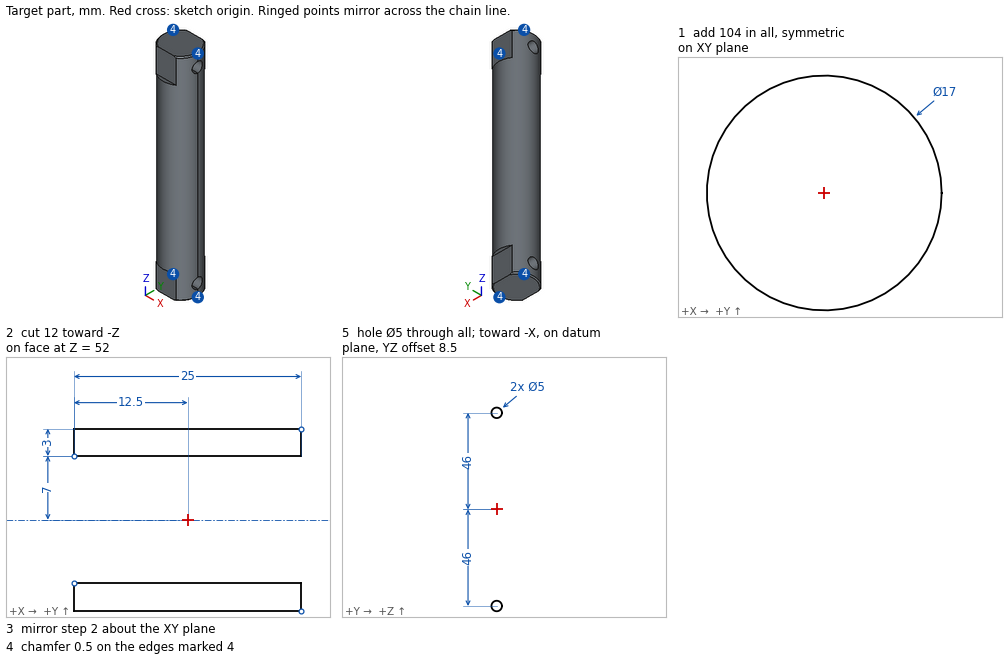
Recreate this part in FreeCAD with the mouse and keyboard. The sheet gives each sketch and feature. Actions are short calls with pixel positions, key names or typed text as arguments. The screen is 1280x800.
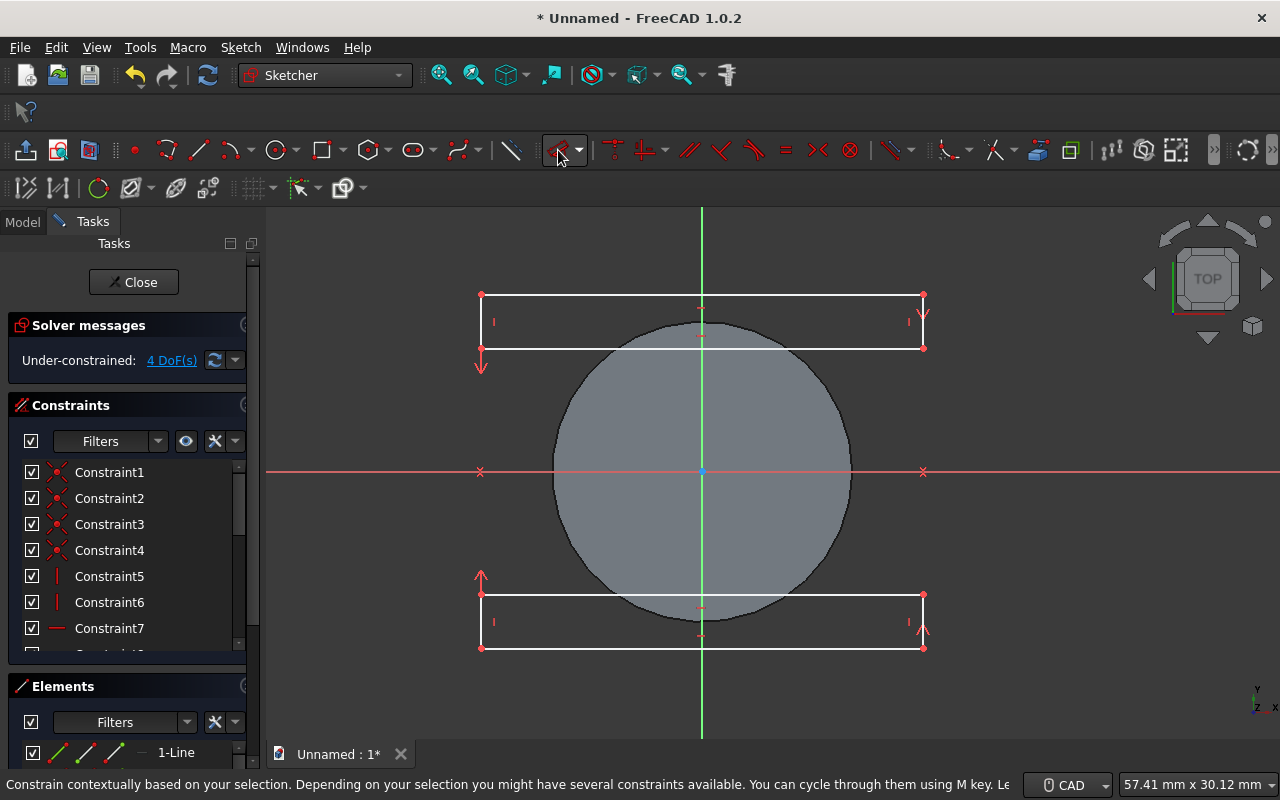
click(481, 311)
click(447, 322)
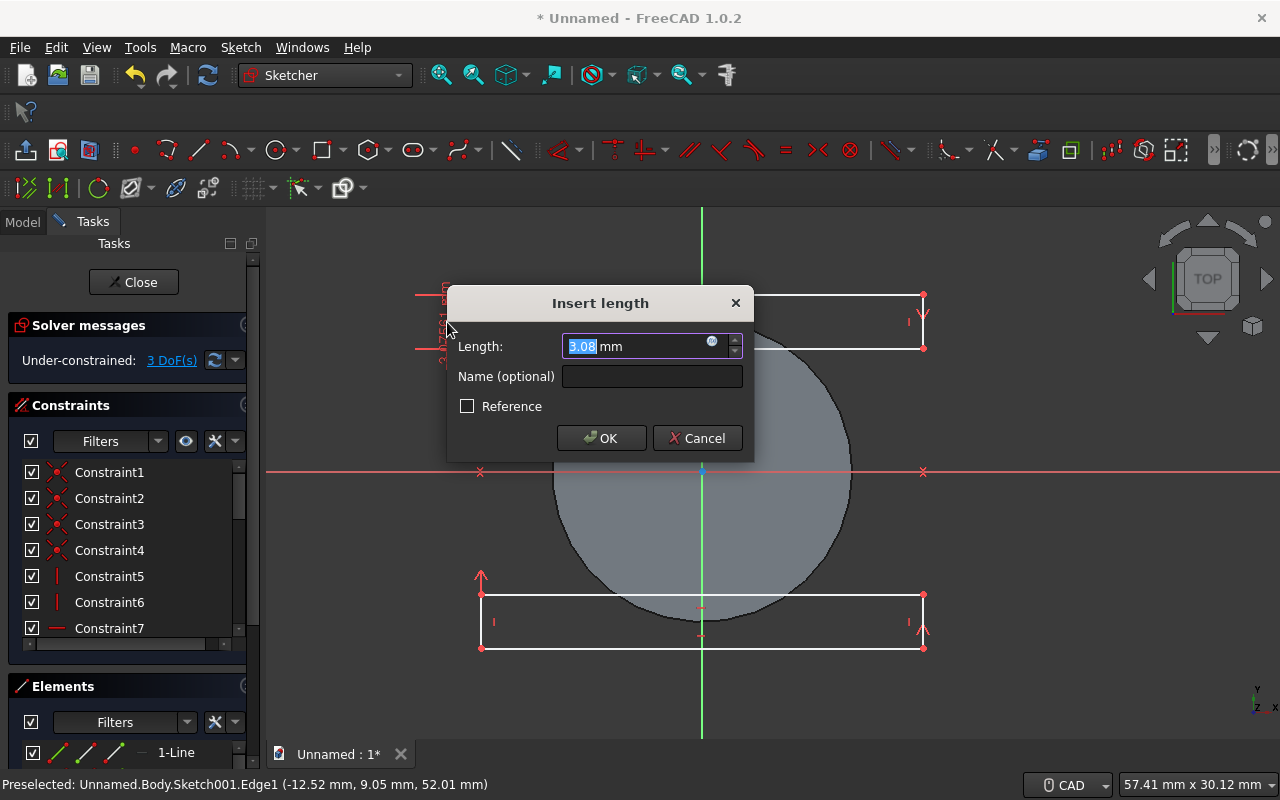
text(3)
key(Return)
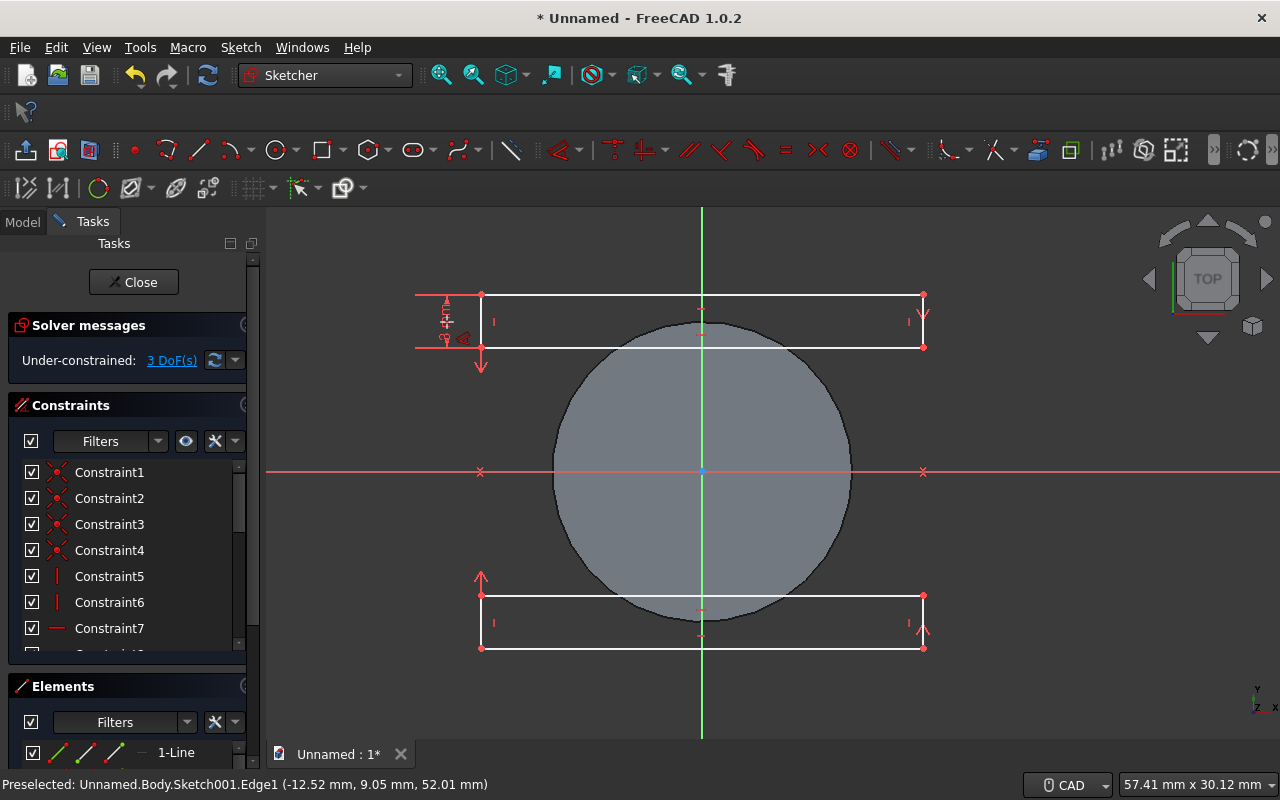
click(614, 348)
click(600, 314)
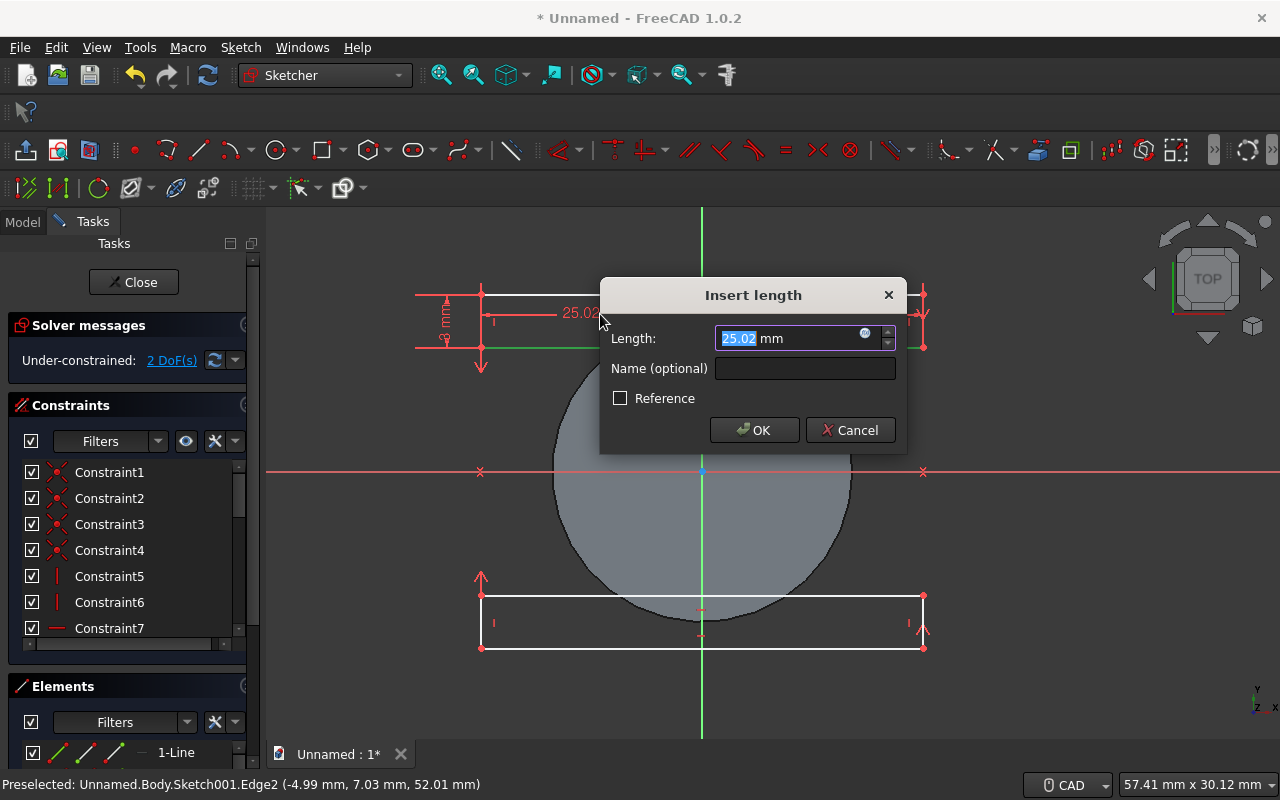
text(25)
key(Return)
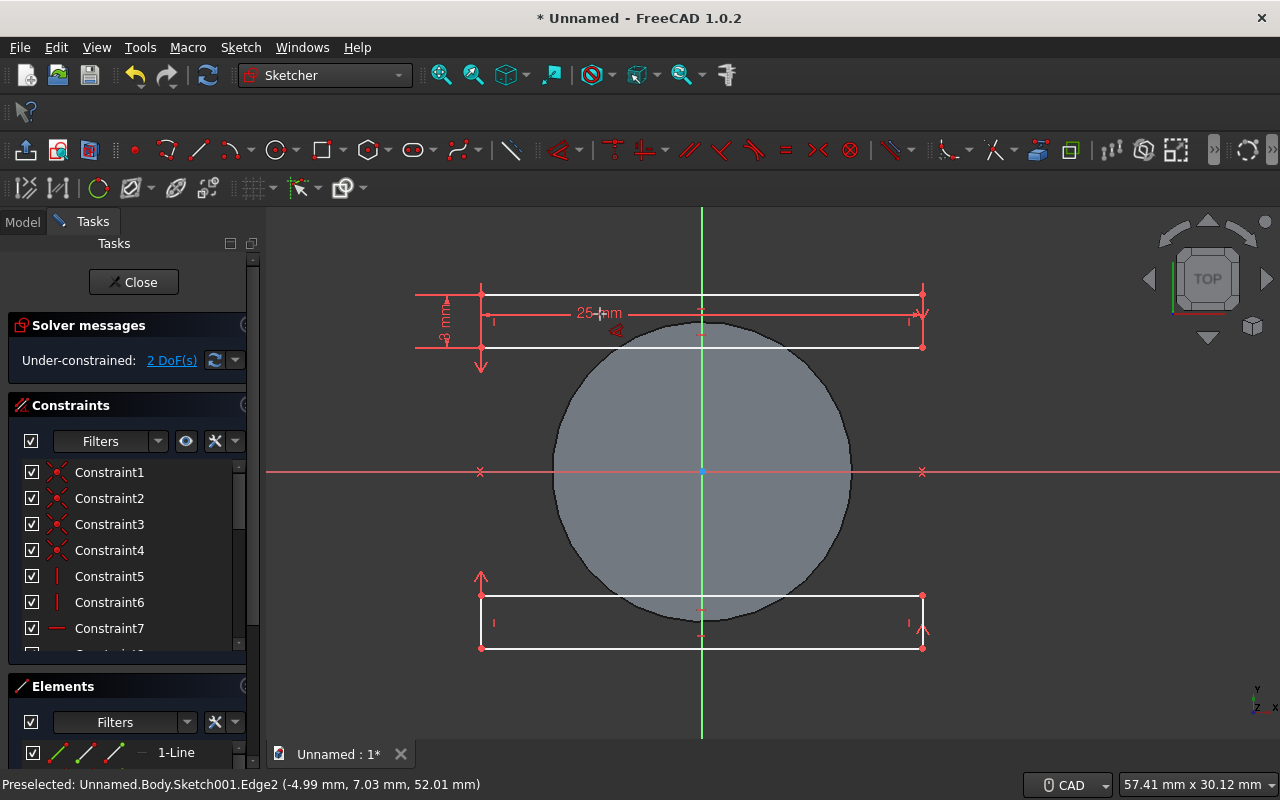
click(481, 348)
click(447, 410)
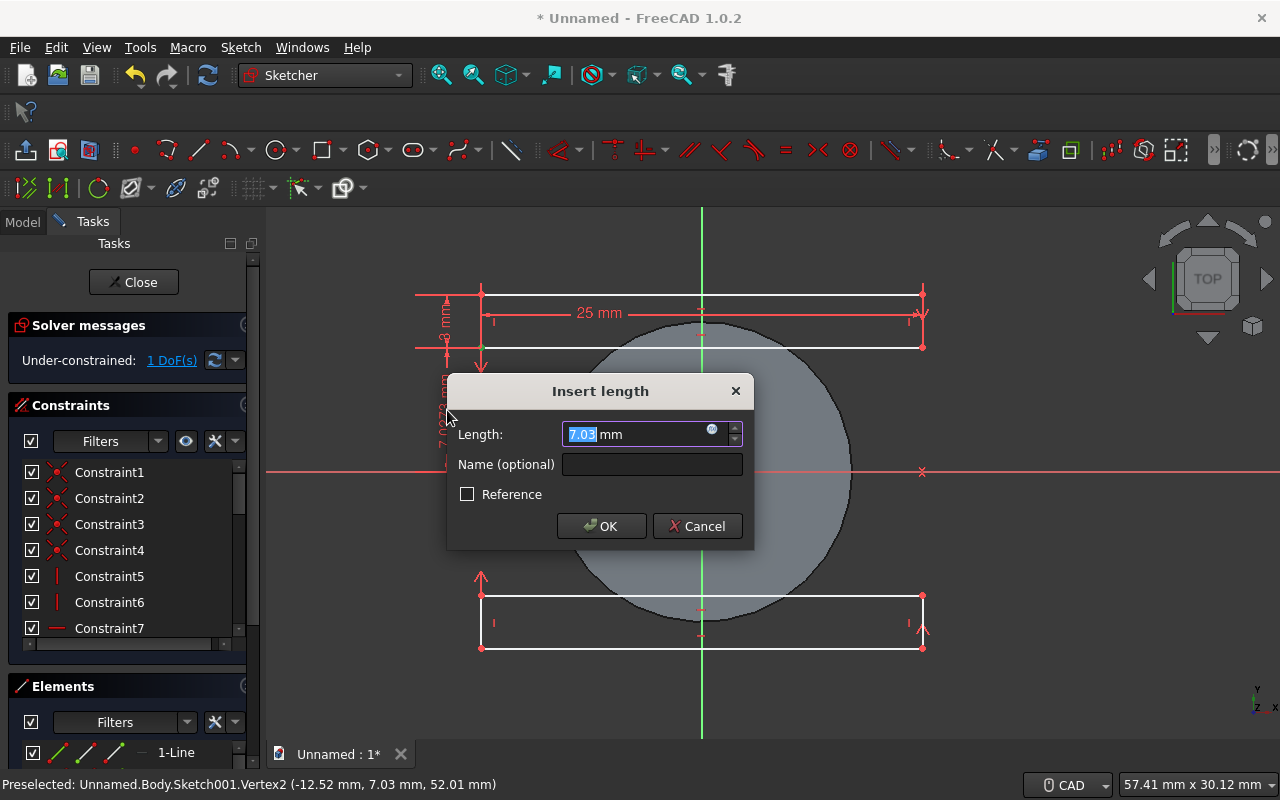
text(7)
key(Return)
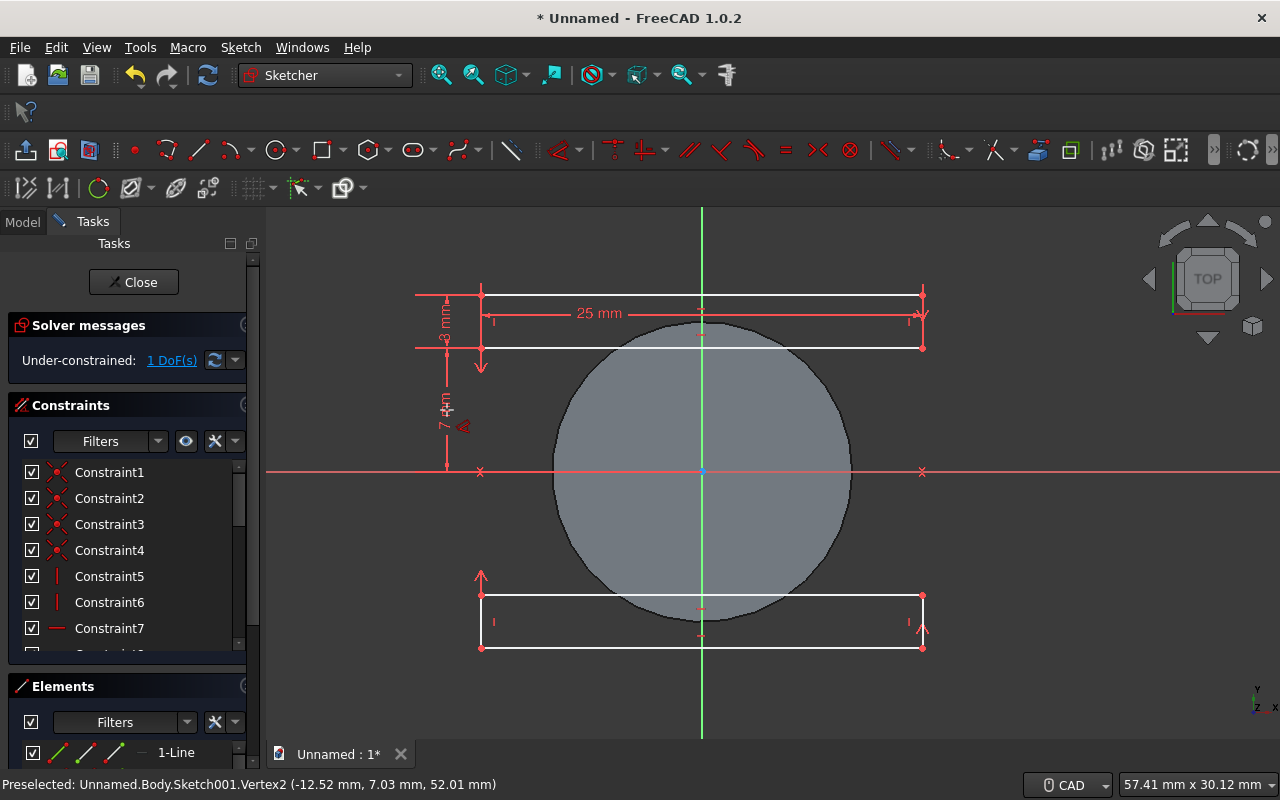
click(481, 295)
click(592, 261)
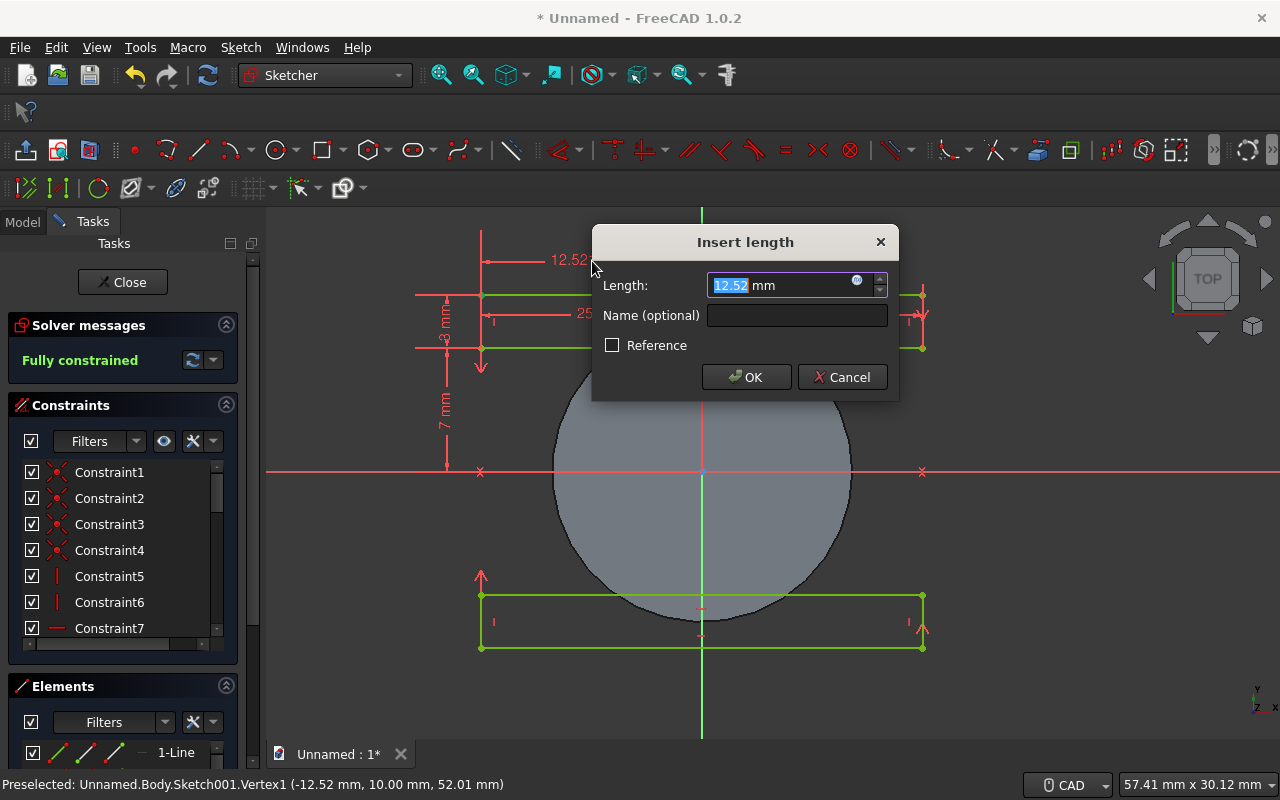
text(12.5)
key(Return)
key(Escape)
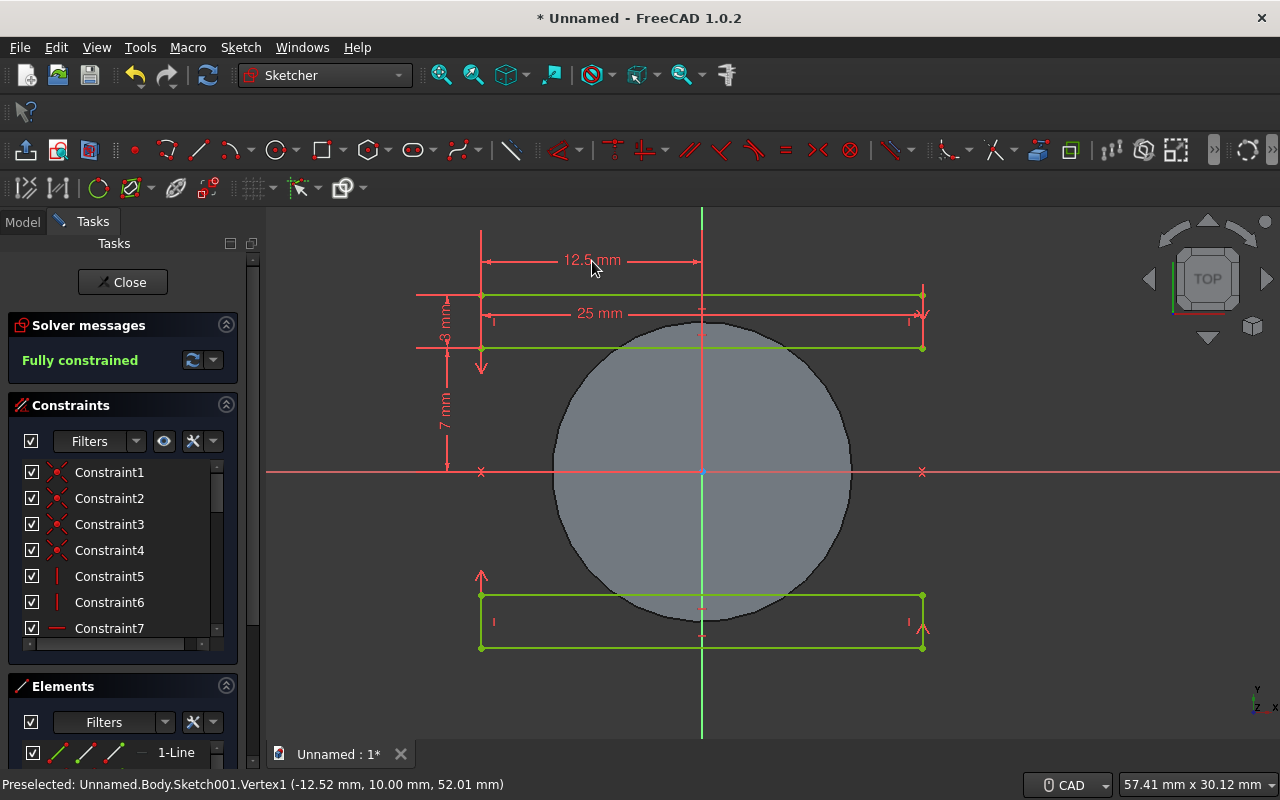
click(123, 282)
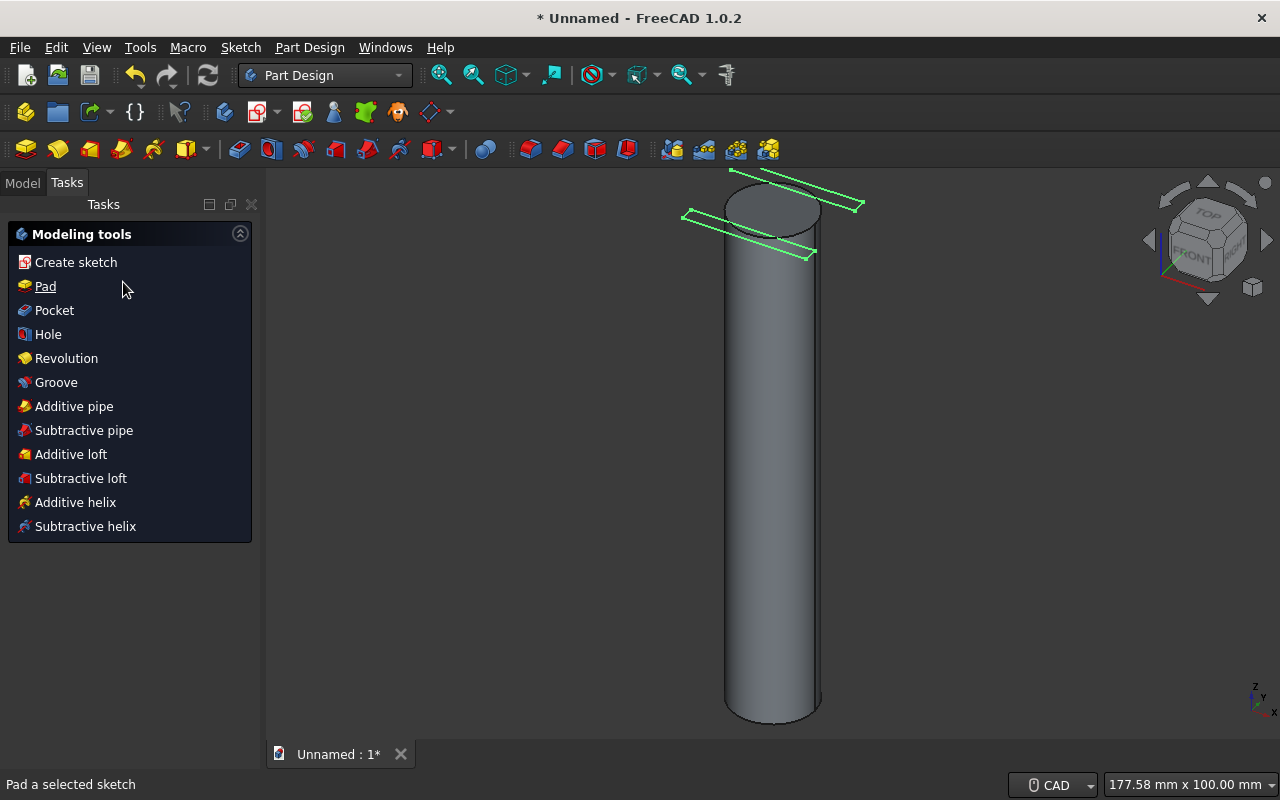
click(240, 150)